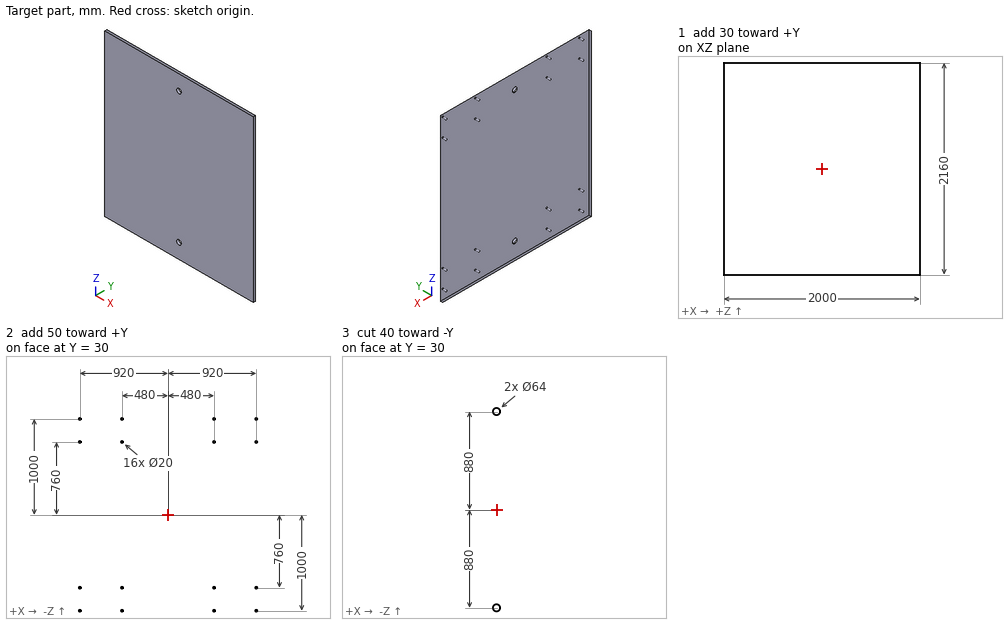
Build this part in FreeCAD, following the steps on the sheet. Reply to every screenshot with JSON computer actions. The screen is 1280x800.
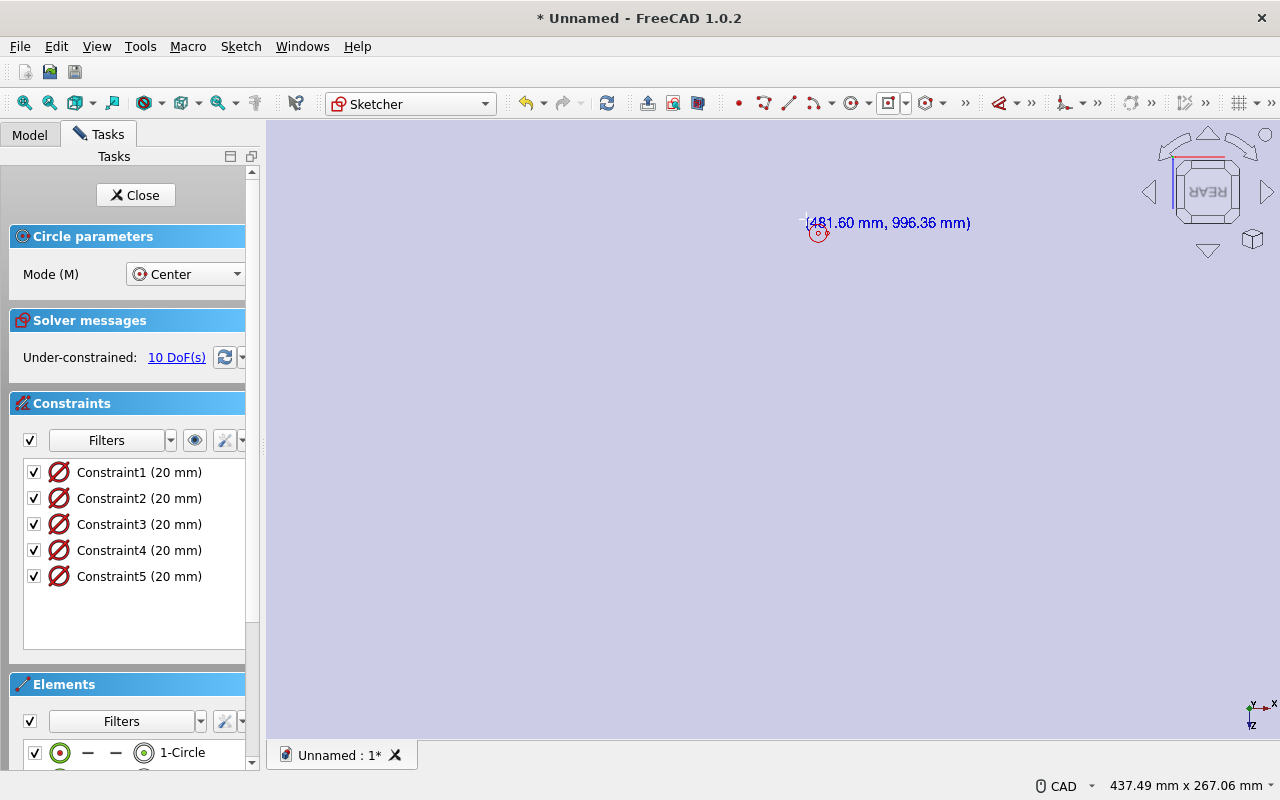
{"action": "scroll", "coordinate": [806, 219], "scroll_direction": "down", "scroll_amount": 12}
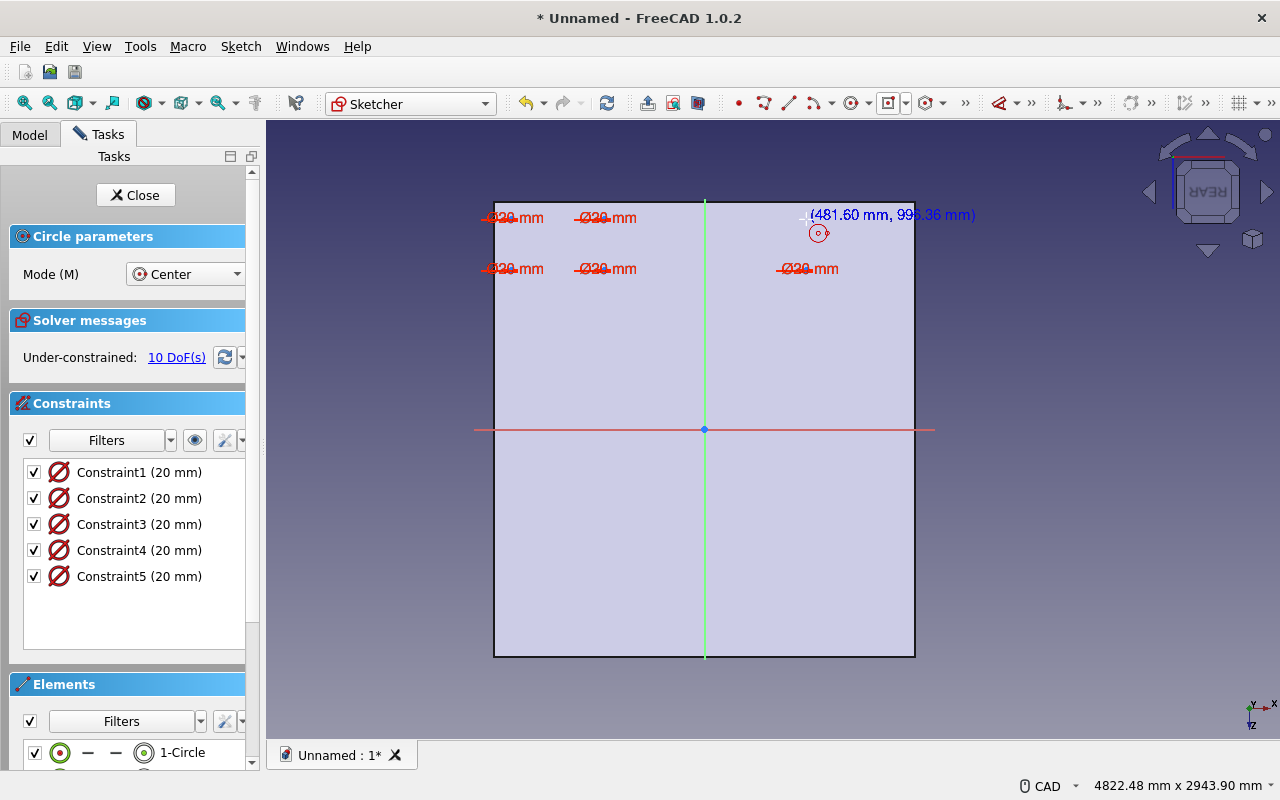
{"action": "left_click", "coordinate": [806, 219]}
{"action": "mouse_move", "coordinate": [807, 218]}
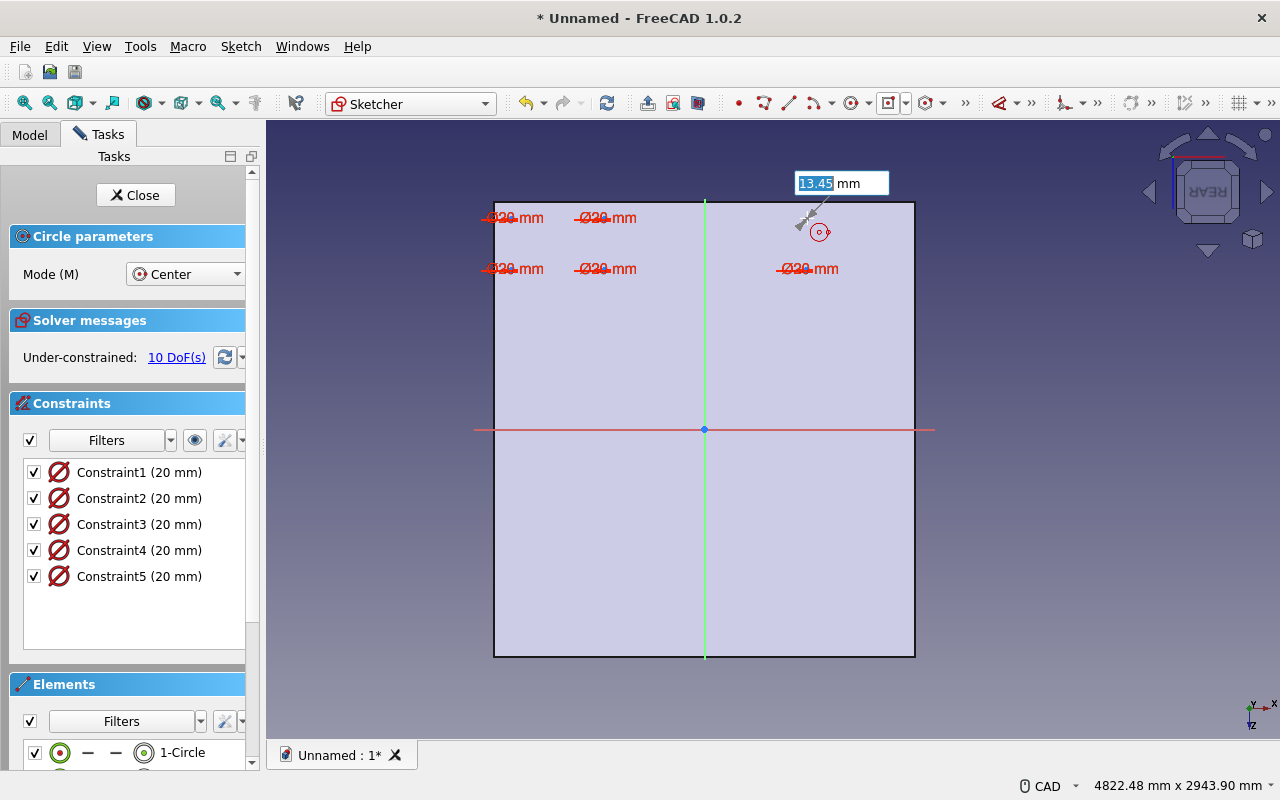
{"action": "type", "text": "20"}
{"action": "key", "text": "Return"}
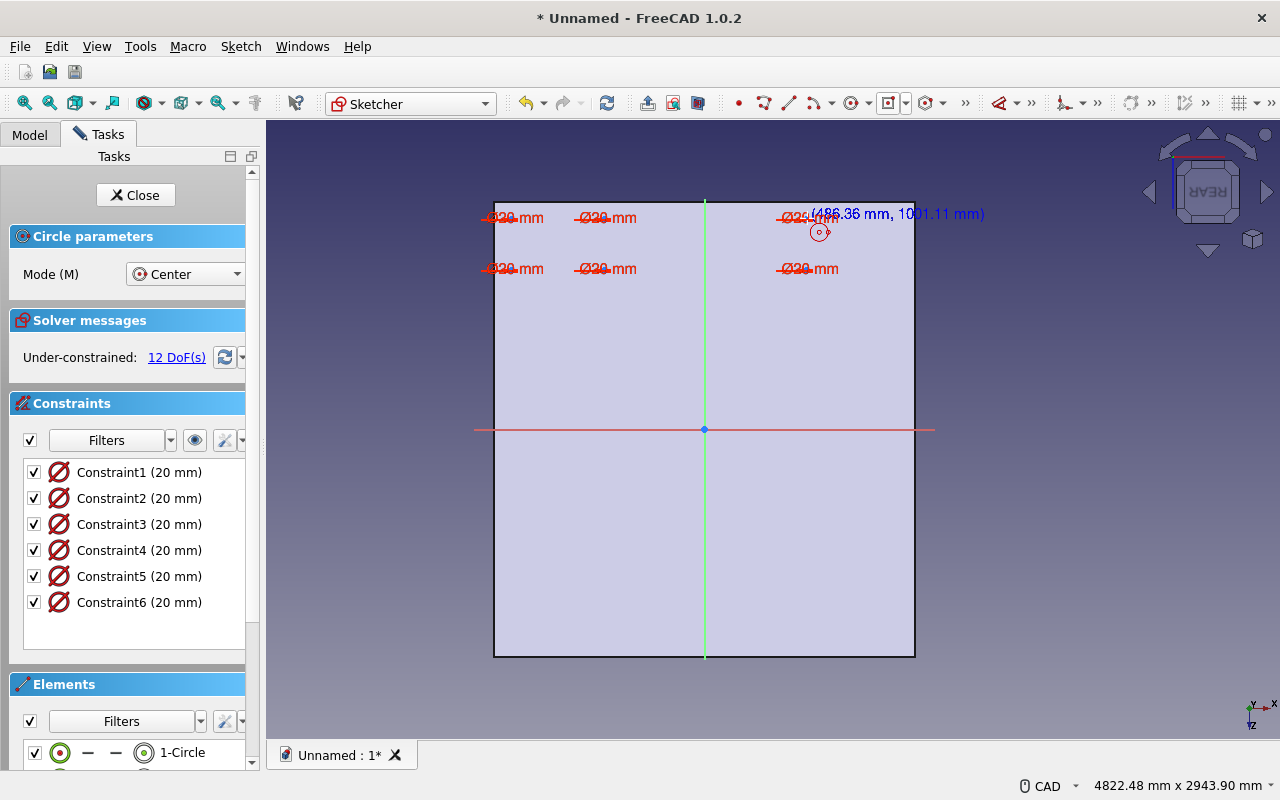
{"action": "scroll", "coordinate": [898, 270], "scroll_direction": "up", "scroll_amount": 12}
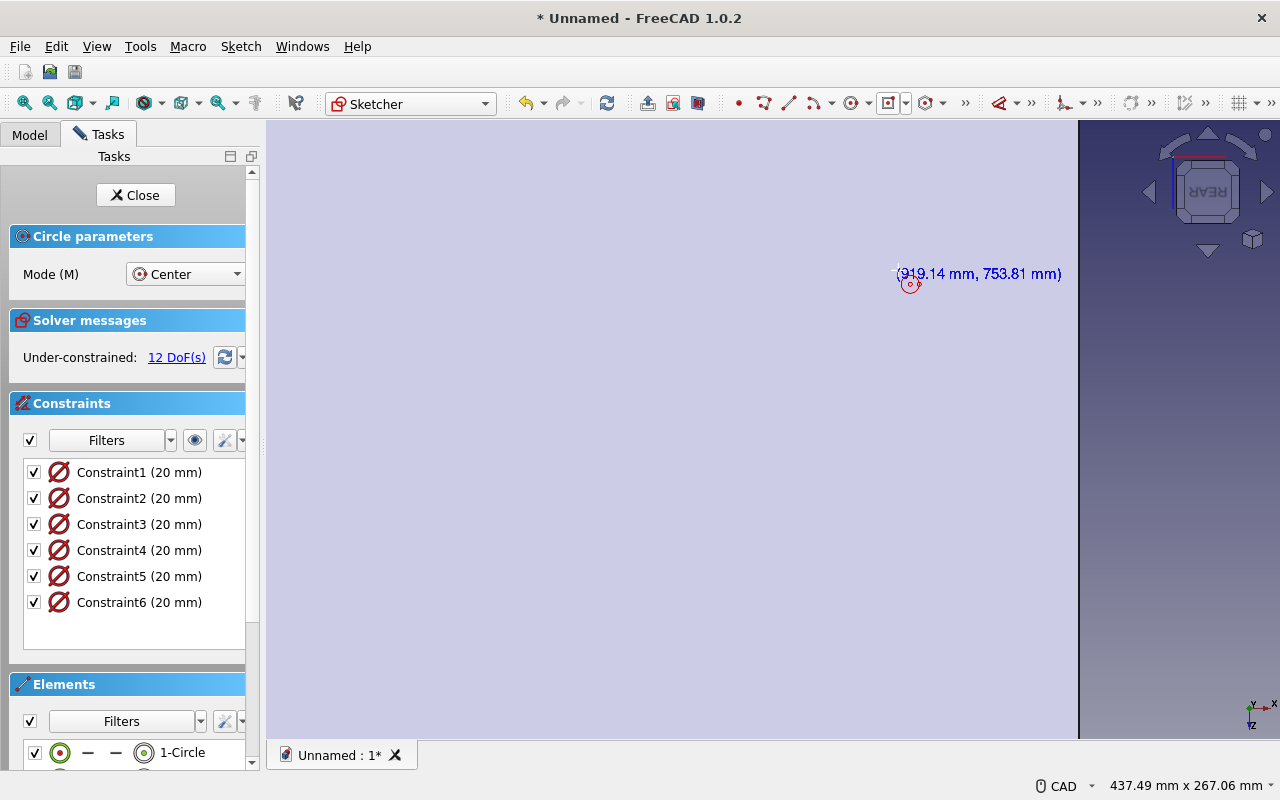
{"action": "scroll", "coordinate": [898, 270], "scroll_direction": "down", "scroll_amount": 12}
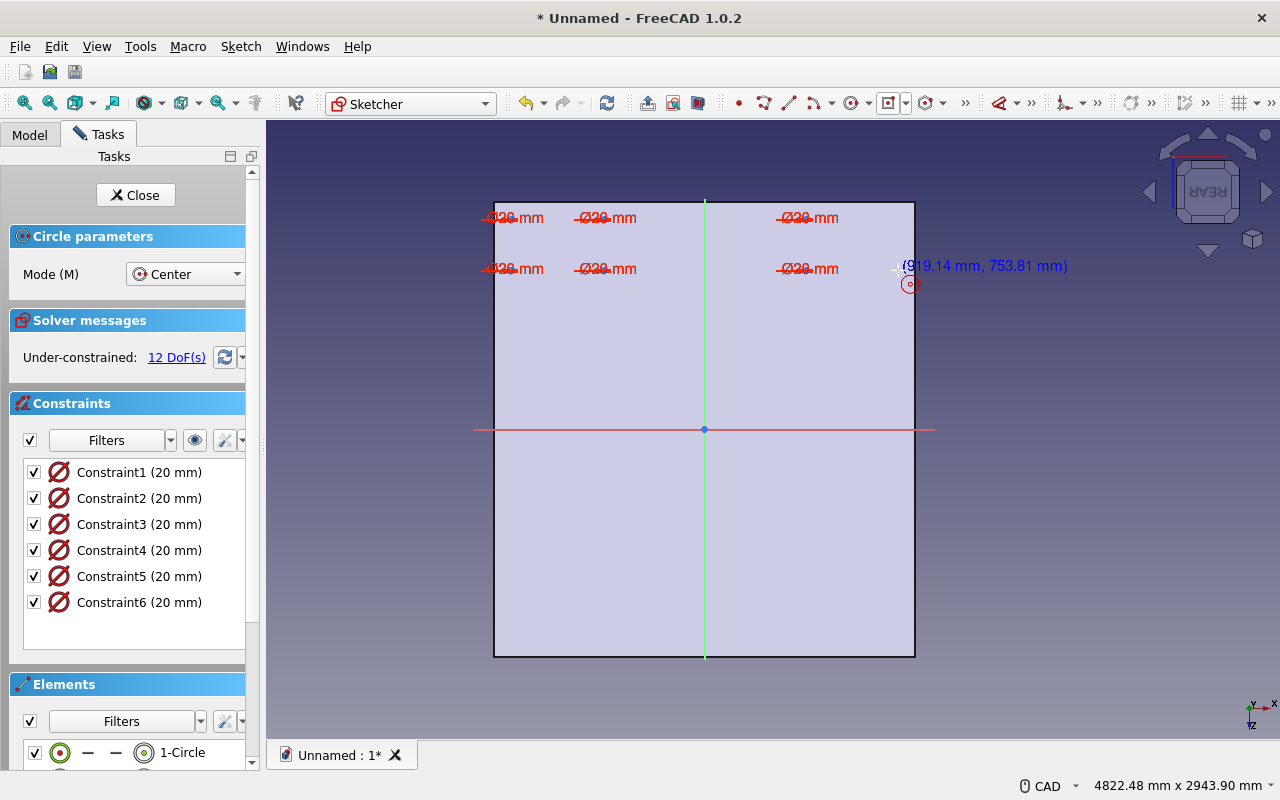
{"action": "left_click", "coordinate": [898, 270]}
{"action": "mouse_move", "coordinate": [900, 268]}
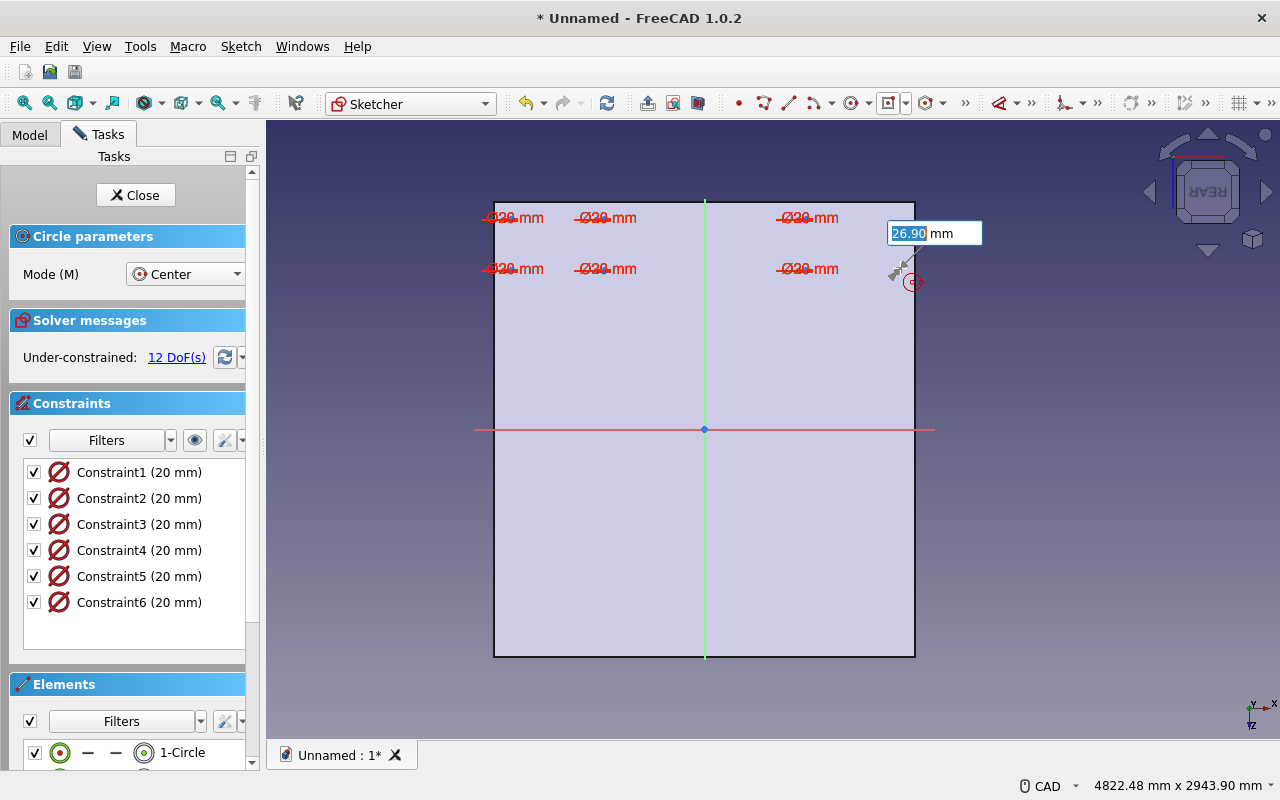
{"action": "type", "text": "20"}
{"action": "key", "text": "Return"}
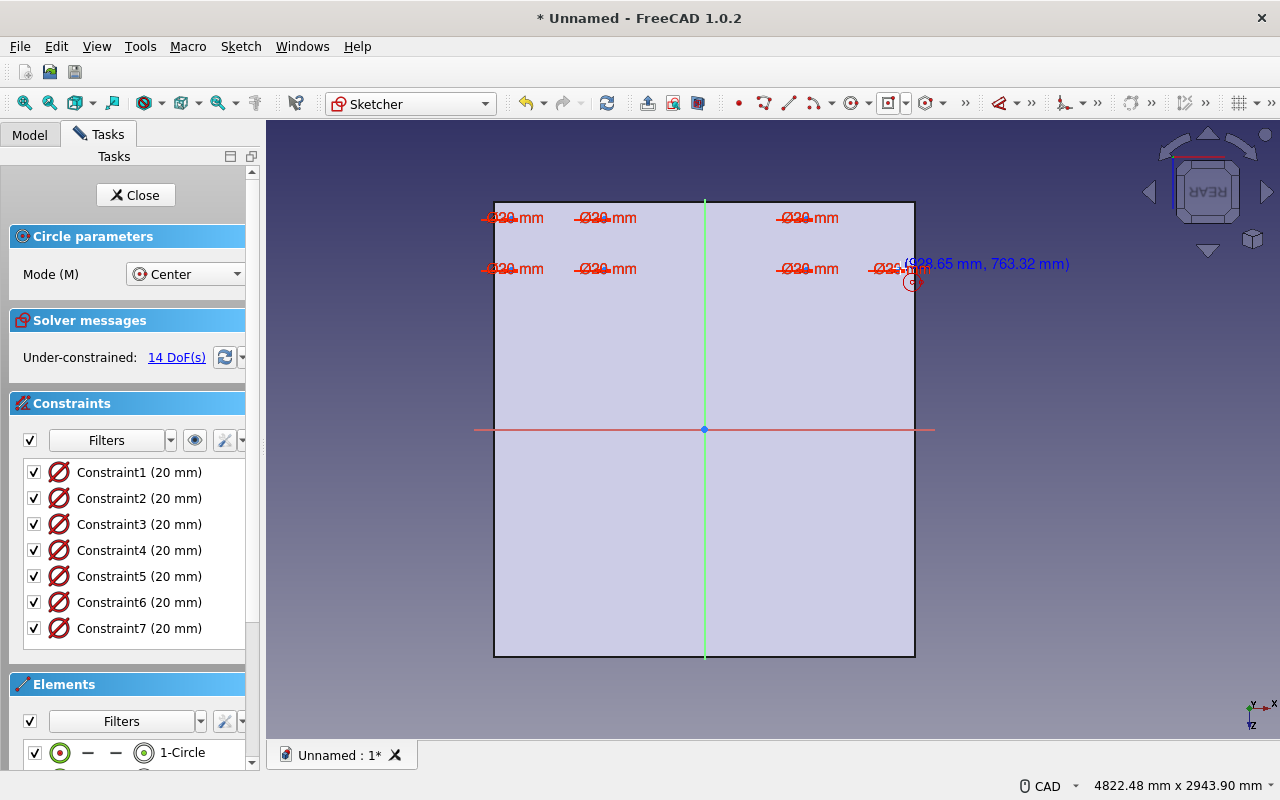
{"action": "scroll", "coordinate": [898, 219], "scroll_direction": "up", "scroll_amount": 12}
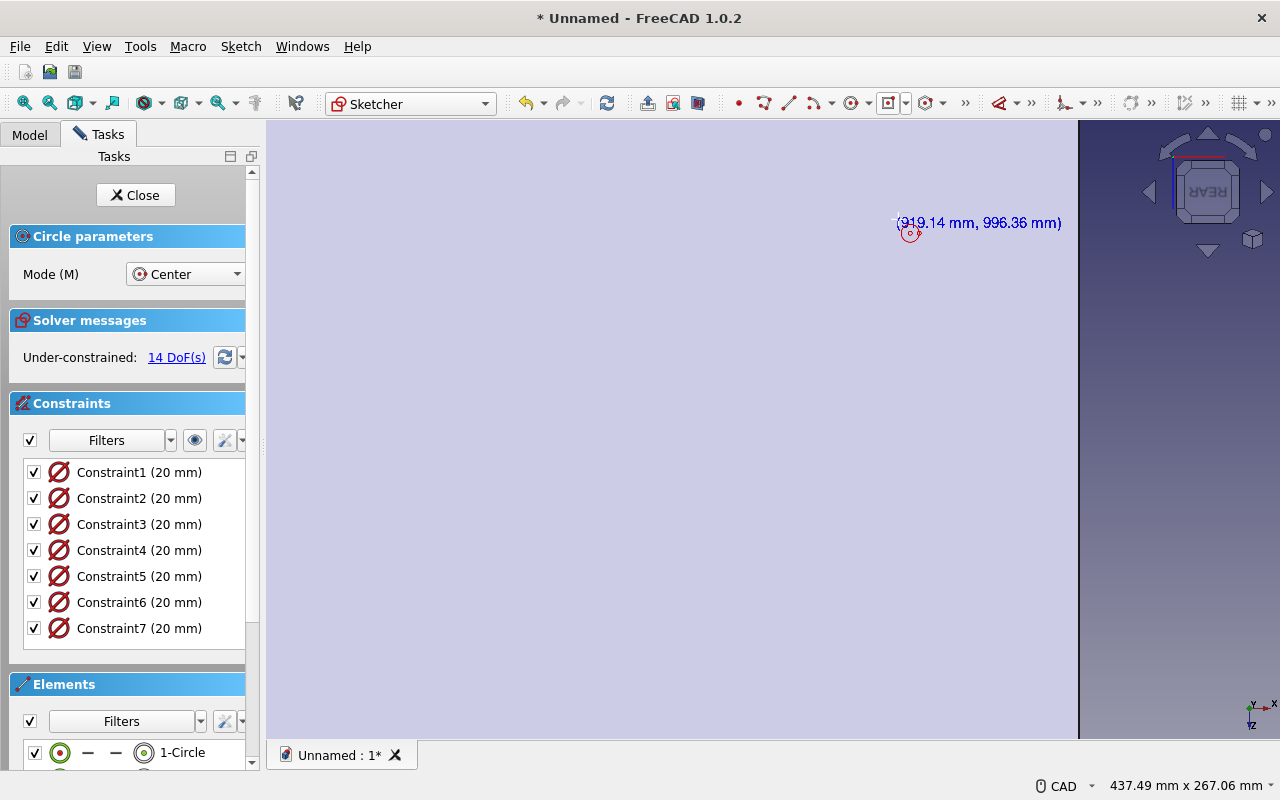
{"action": "scroll", "coordinate": [898, 219], "scroll_direction": "down", "scroll_amount": 12}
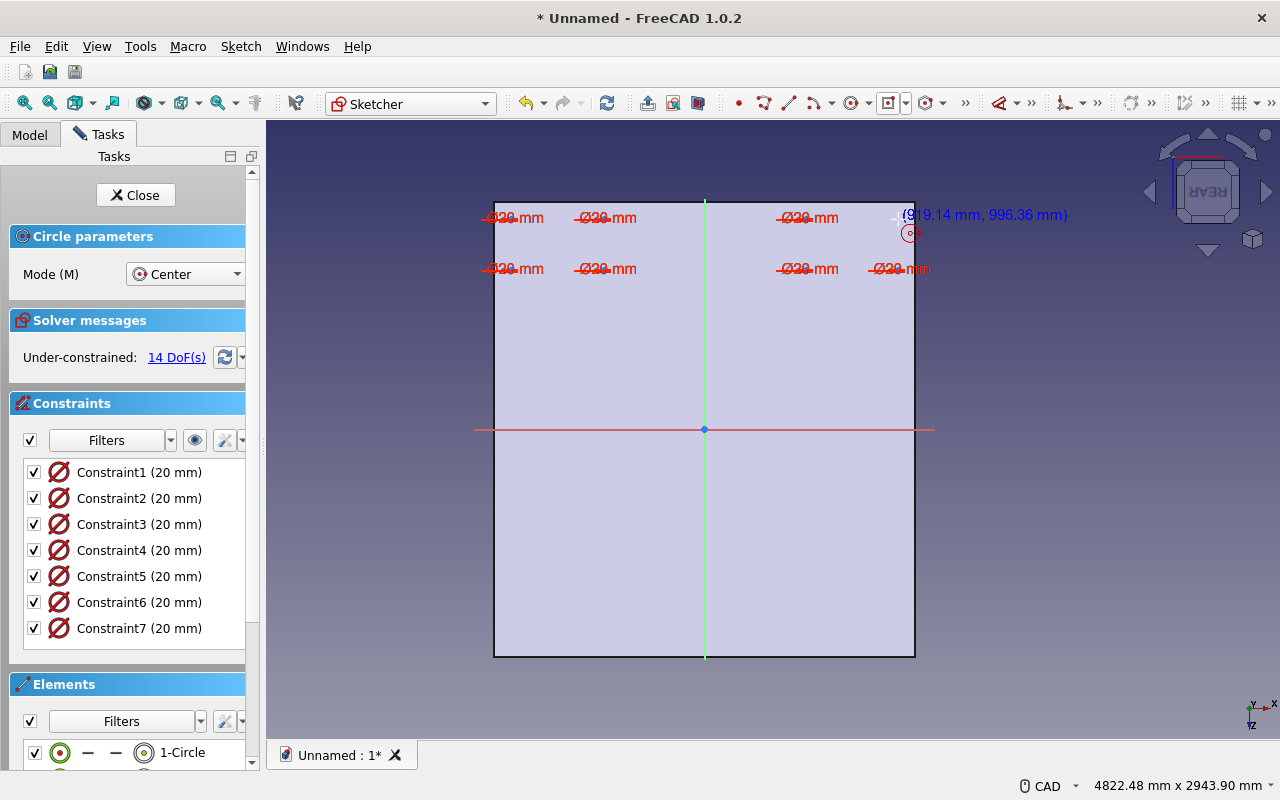
{"action": "left_click", "coordinate": [898, 219]}
{"action": "mouse_move", "coordinate": [900, 218]}